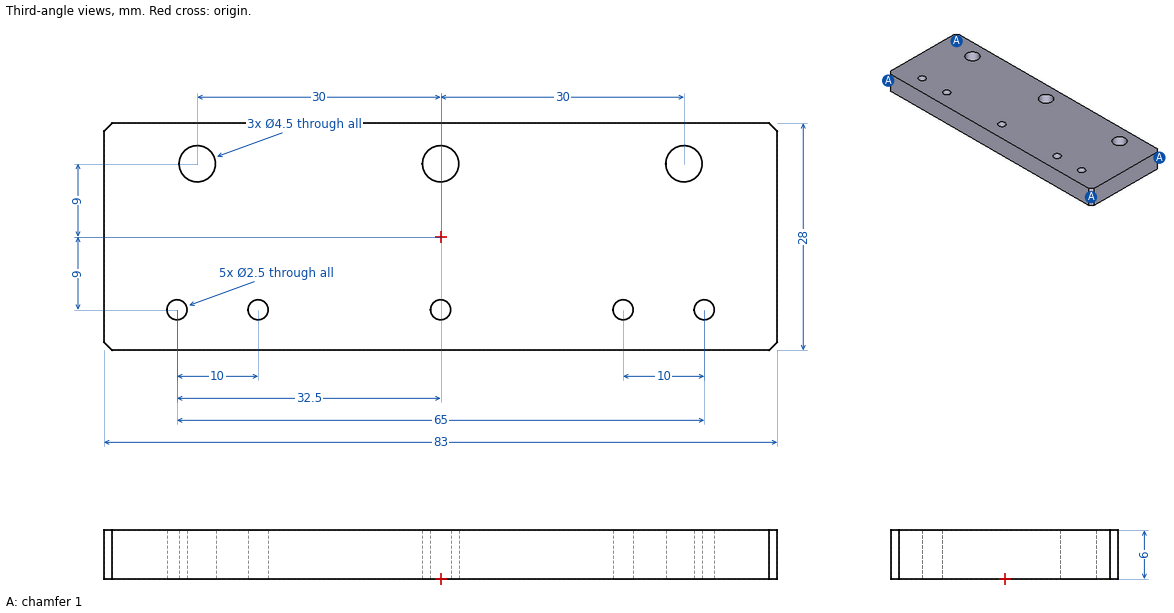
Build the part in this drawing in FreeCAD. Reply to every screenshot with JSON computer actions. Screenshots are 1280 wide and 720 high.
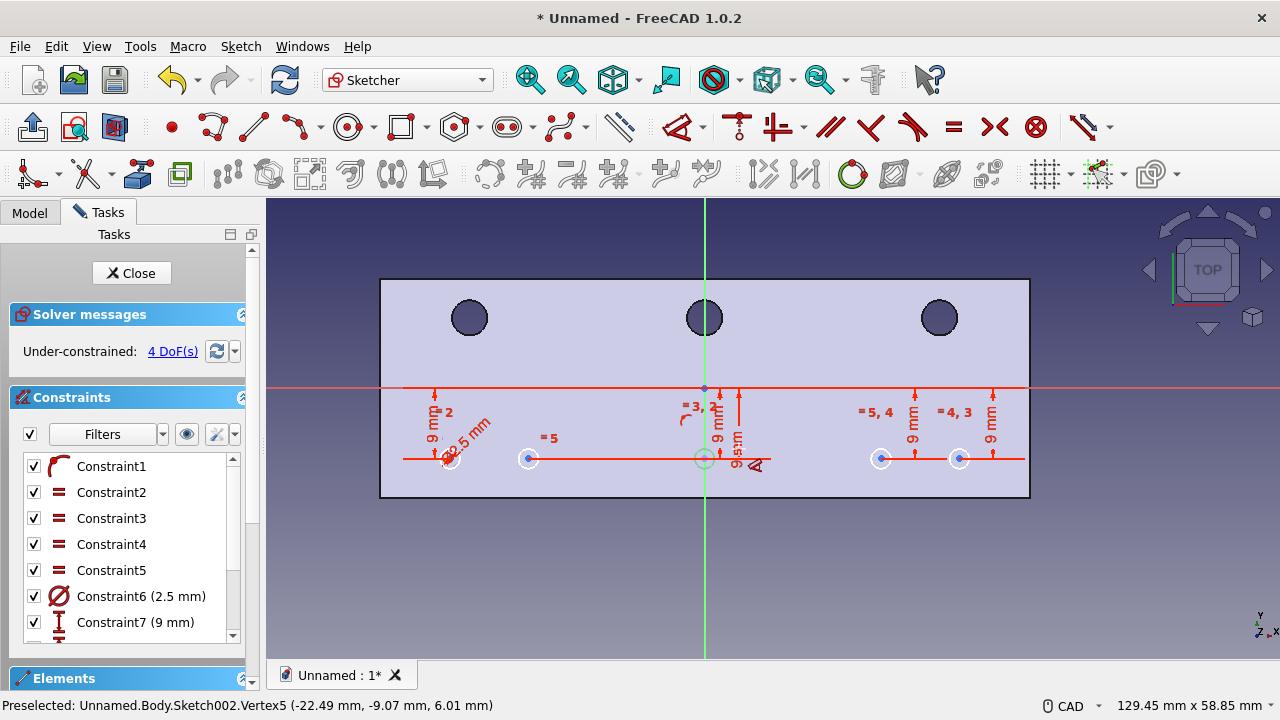
{"action": "left_click", "coordinate": [450, 459]}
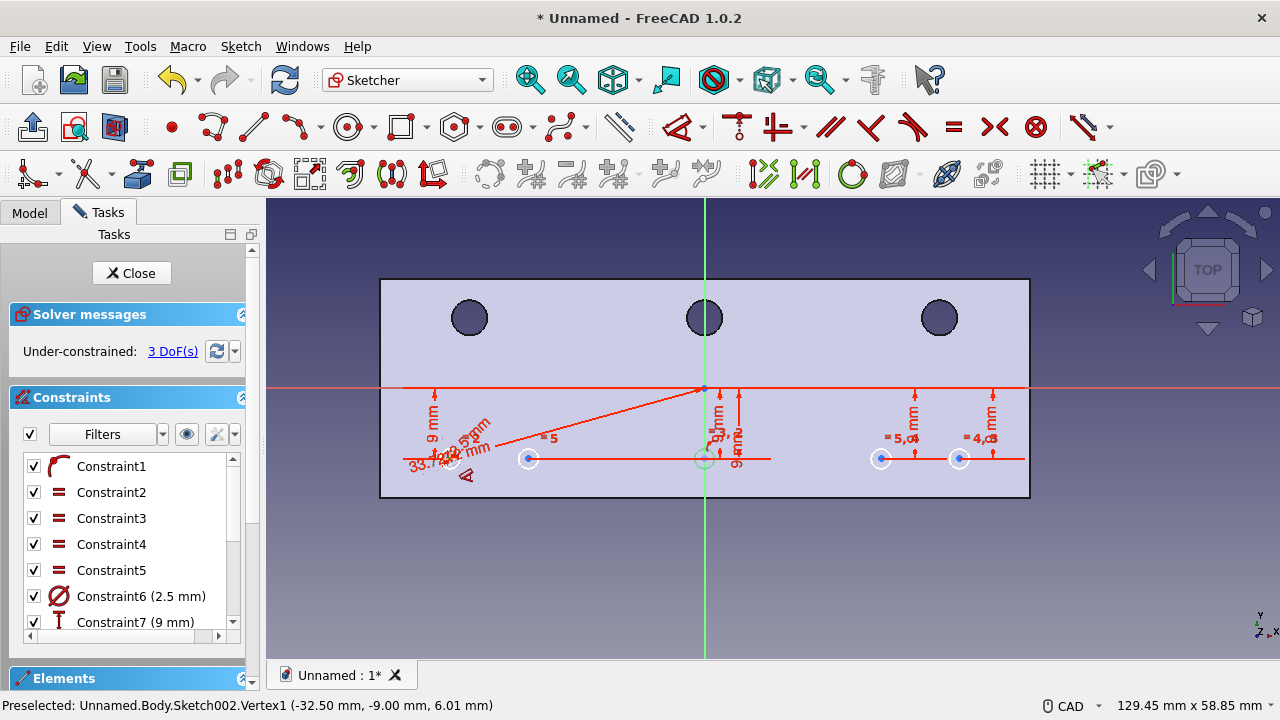
{"action": "left_click", "coordinate": [959, 459]}
{"action": "left_click", "coordinate": [588, 493]}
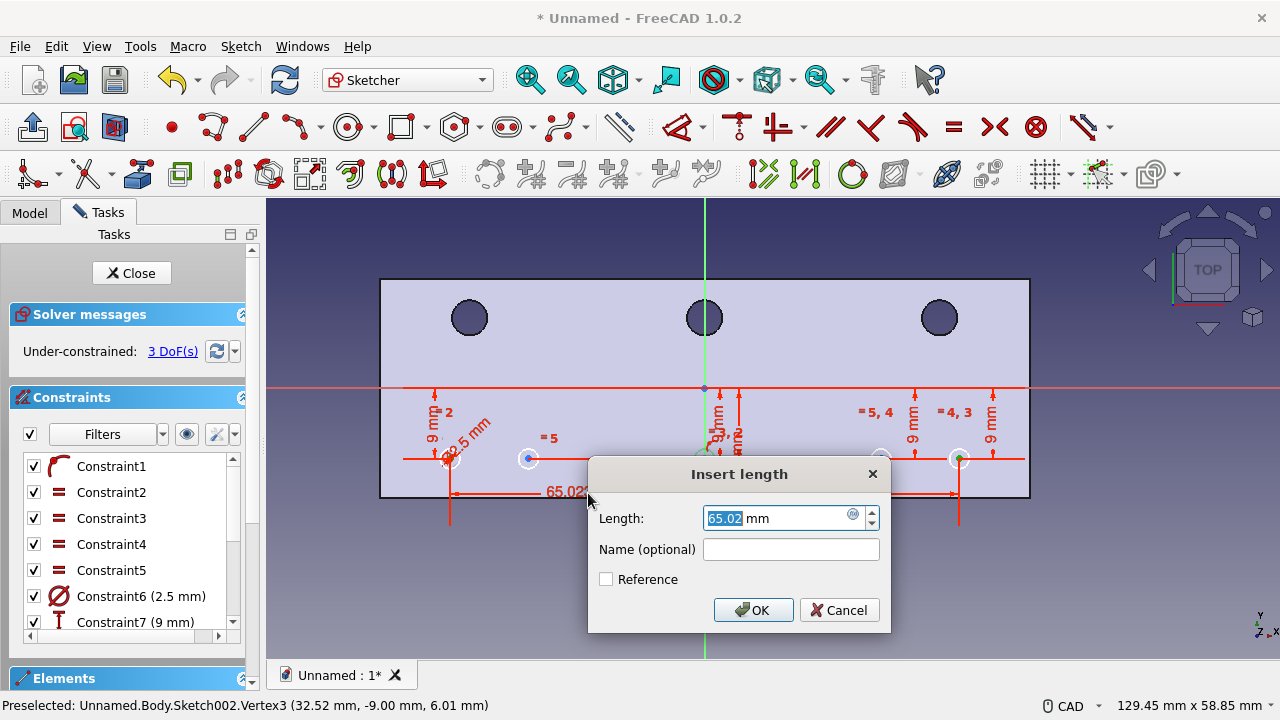
{"action": "type", "text": "65"}
{"action": "key", "text": "Return"}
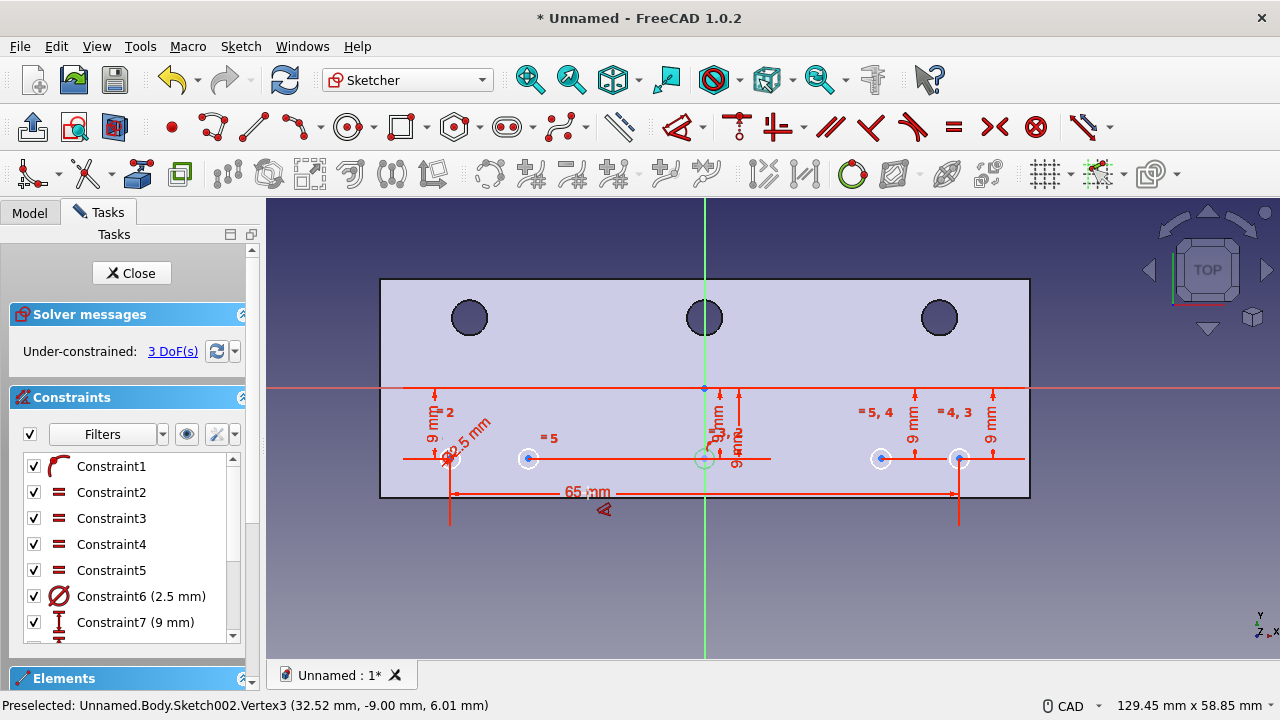
{"action": "left_click", "coordinate": [959, 459]}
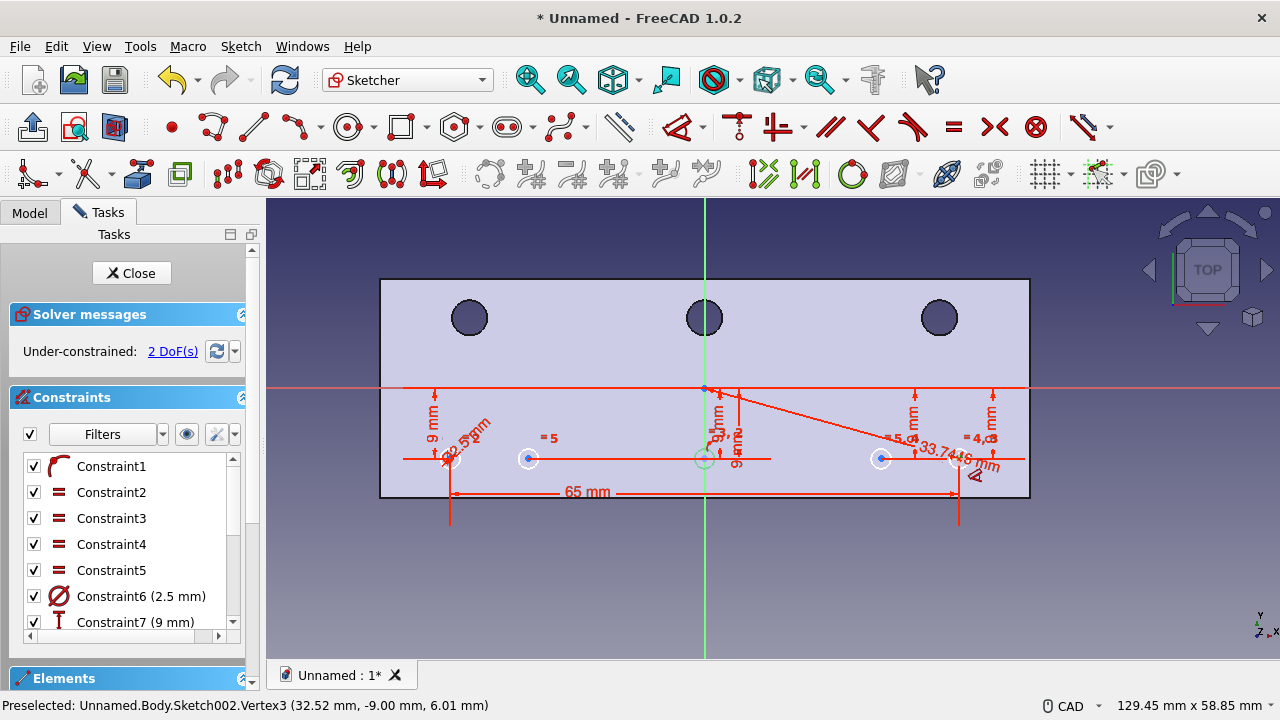
{"action": "left_click", "coordinate": [881, 459]}
{"action": "left_click", "coordinate": [920, 493]}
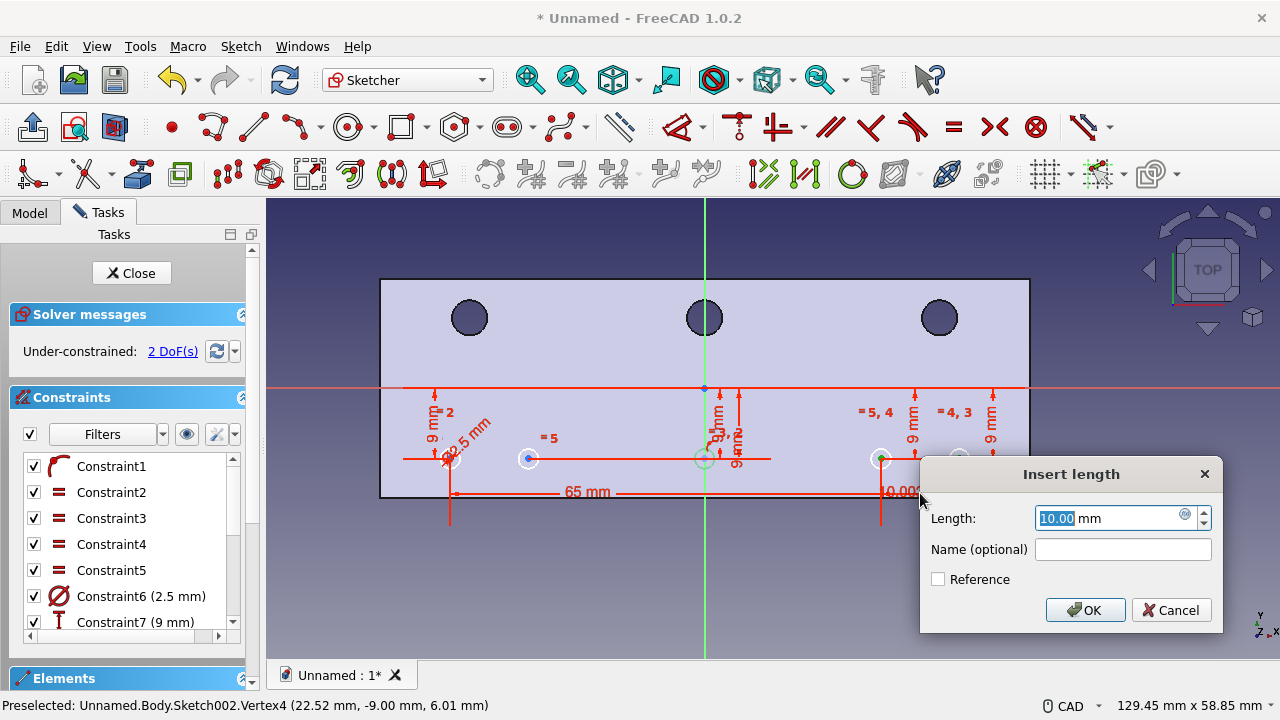
{"action": "type", "text": "10"}
{"action": "key", "text": "Return"}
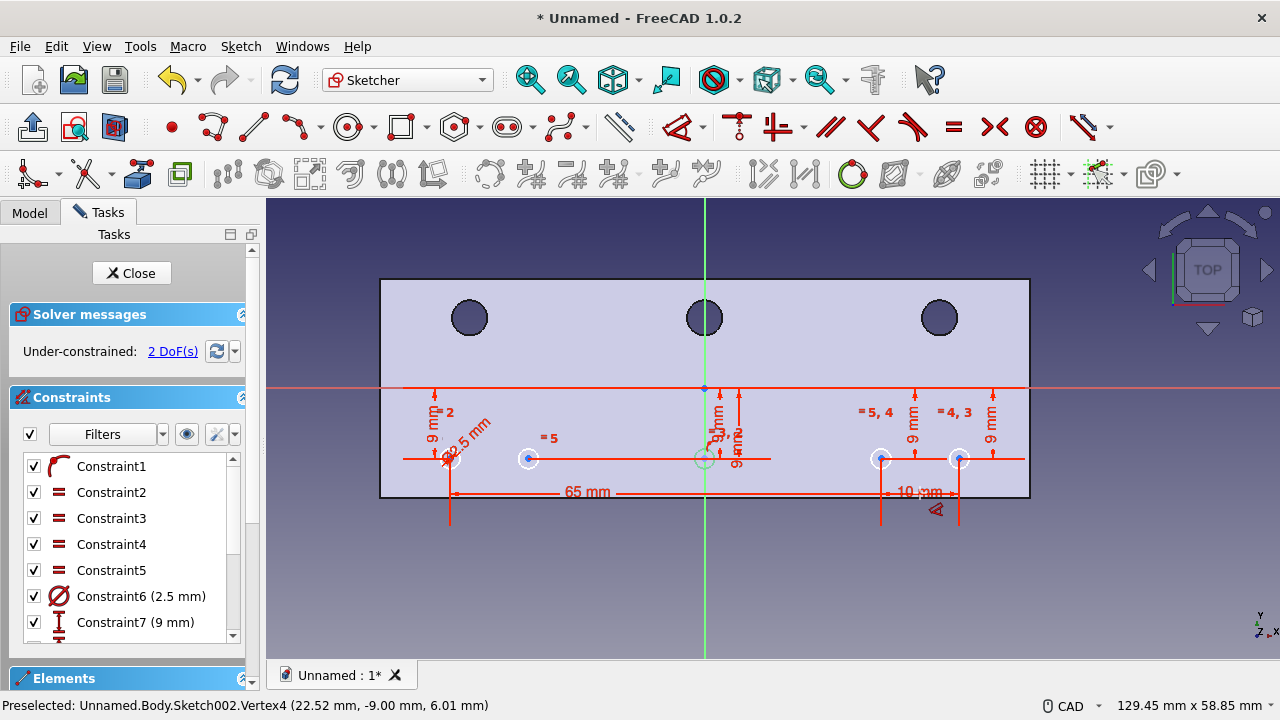
{"action": "left_click", "coordinate": [450, 459]}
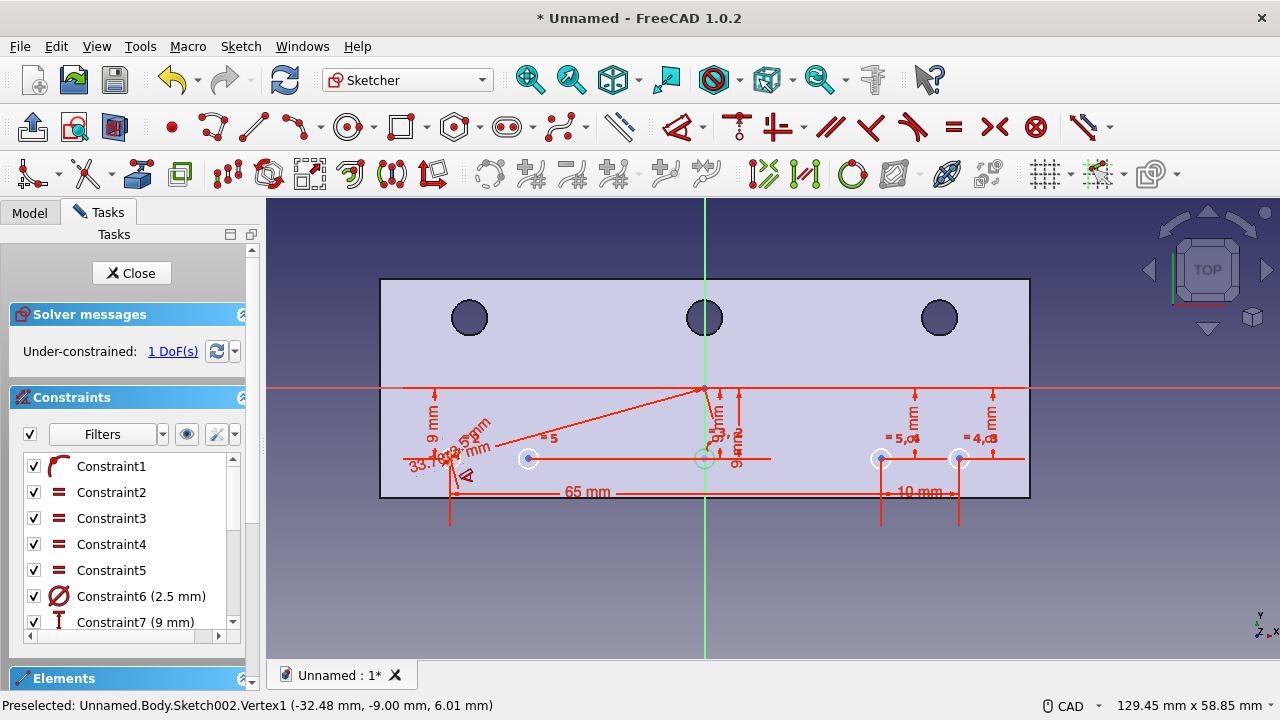
{"action": "left_click", "coordinate": [528, 459]}
{"action": "left_click", "coordinate": [489, 493]}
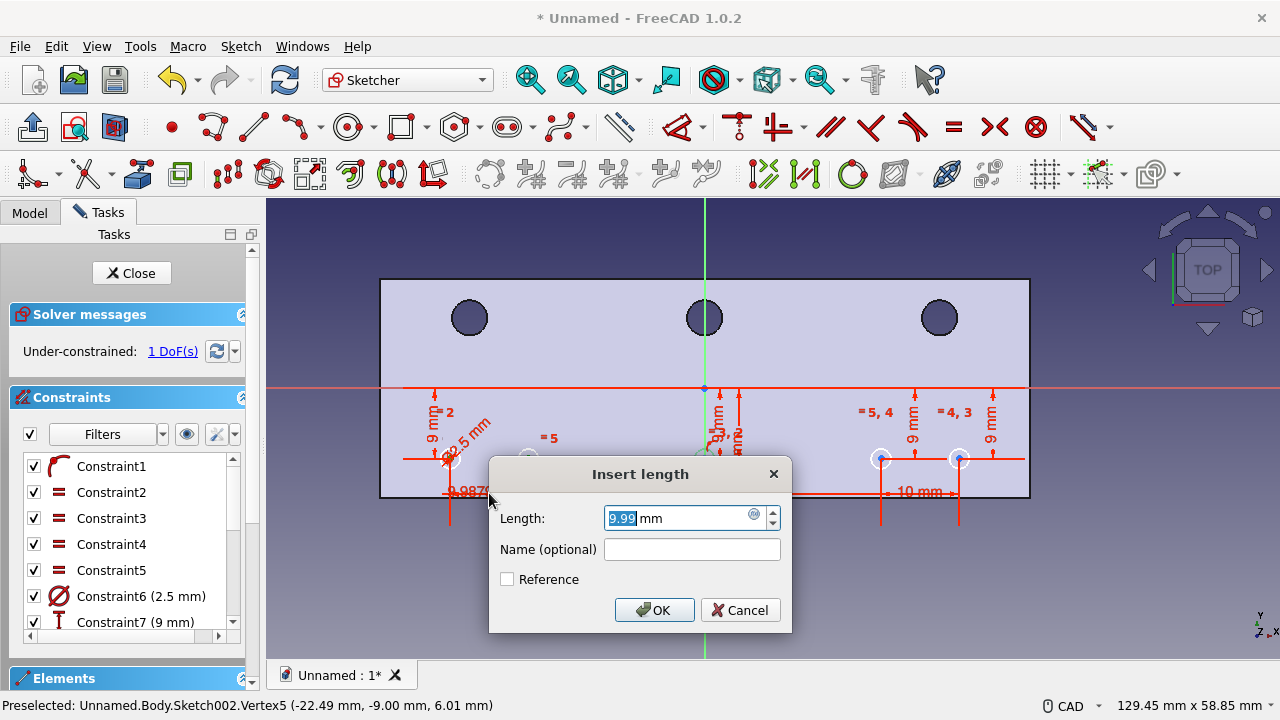
{"action": "type", "text": "10"}
{"action": "key", "text": "Return"}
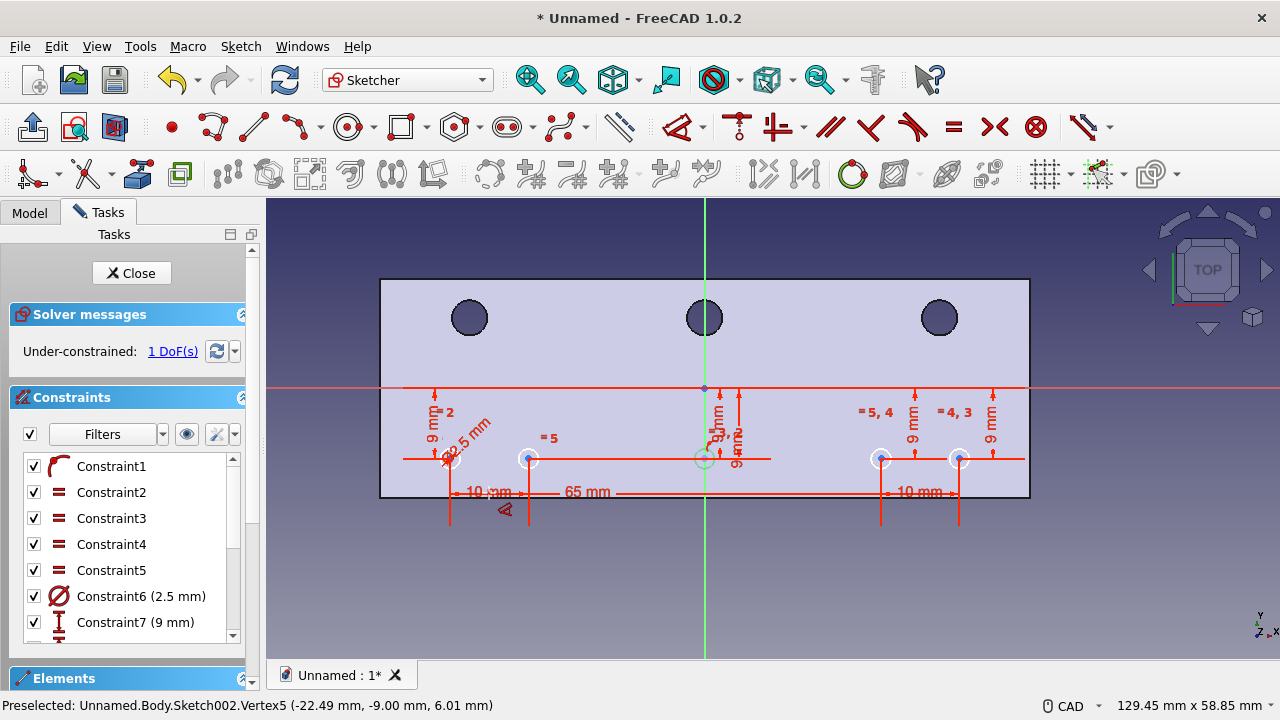
{"action": "left_click", "coordinate": [450, 459]}
{"action": "left_click", "coordinate": [577, 354]}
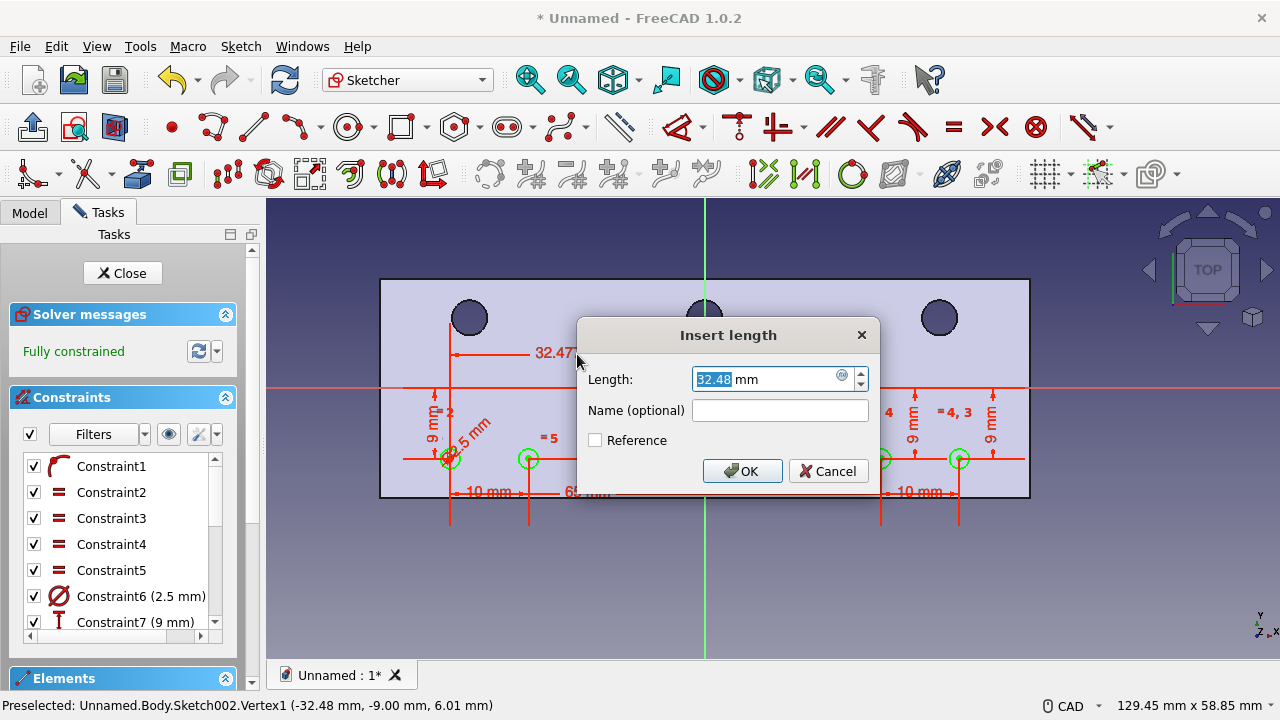
{"action": "type", "text": "32.5"}
{"action": "key", "text": "Return"}
{"action": "key", "text": "Escape"}